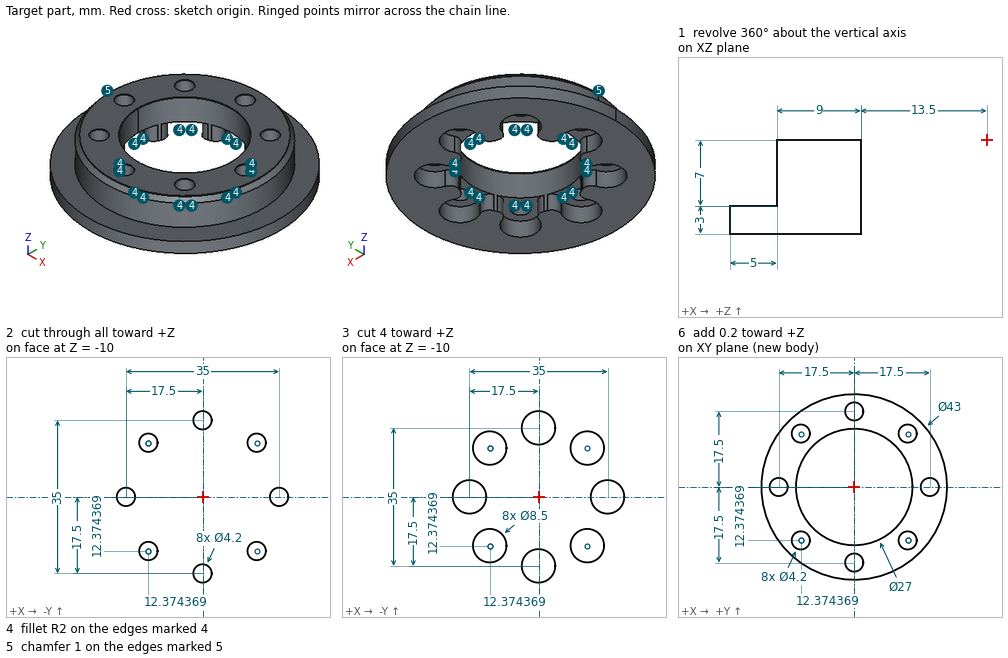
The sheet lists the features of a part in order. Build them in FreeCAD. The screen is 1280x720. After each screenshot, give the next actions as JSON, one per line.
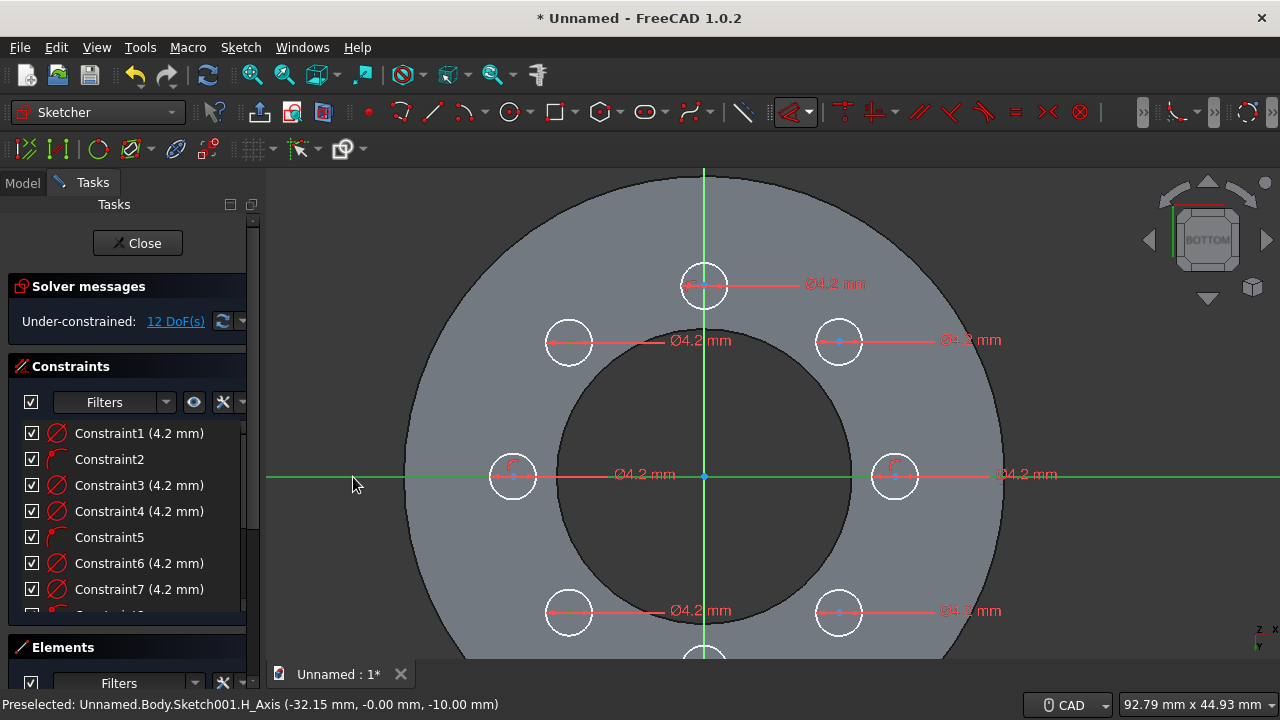
{"action": "key", "text": "s"}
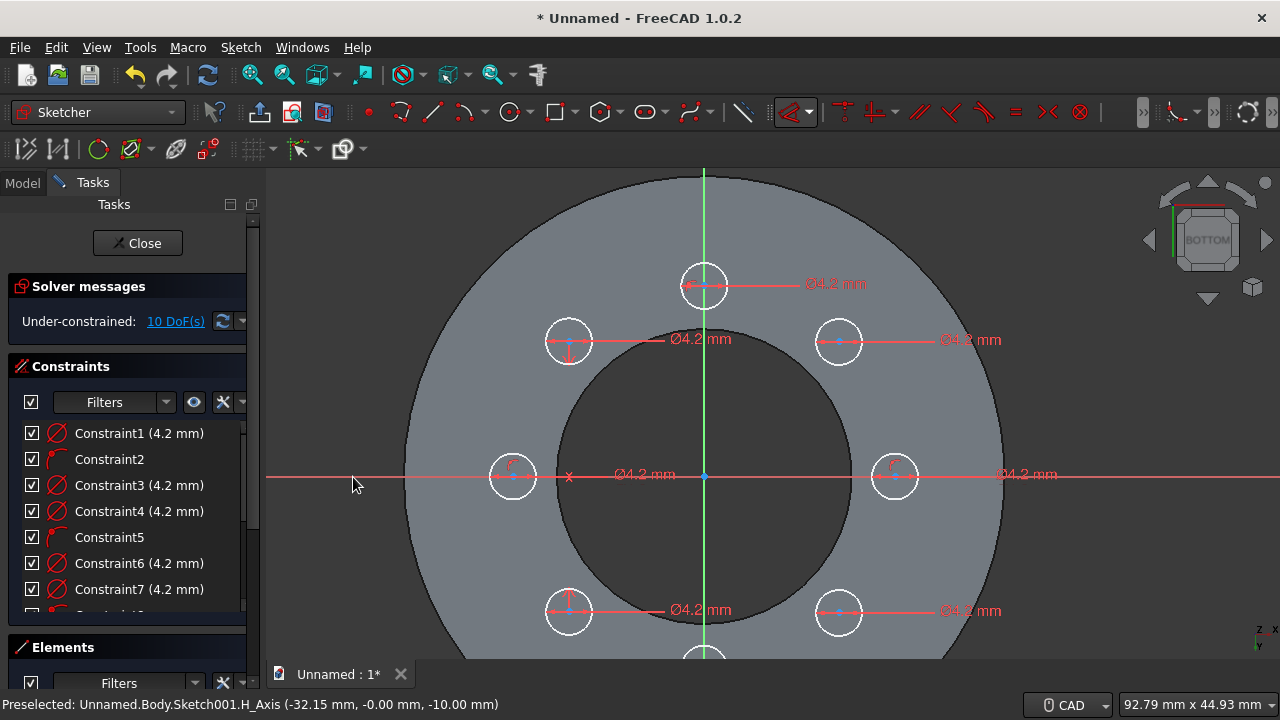
{"action": "left_click", "coordinate": [569, 341]}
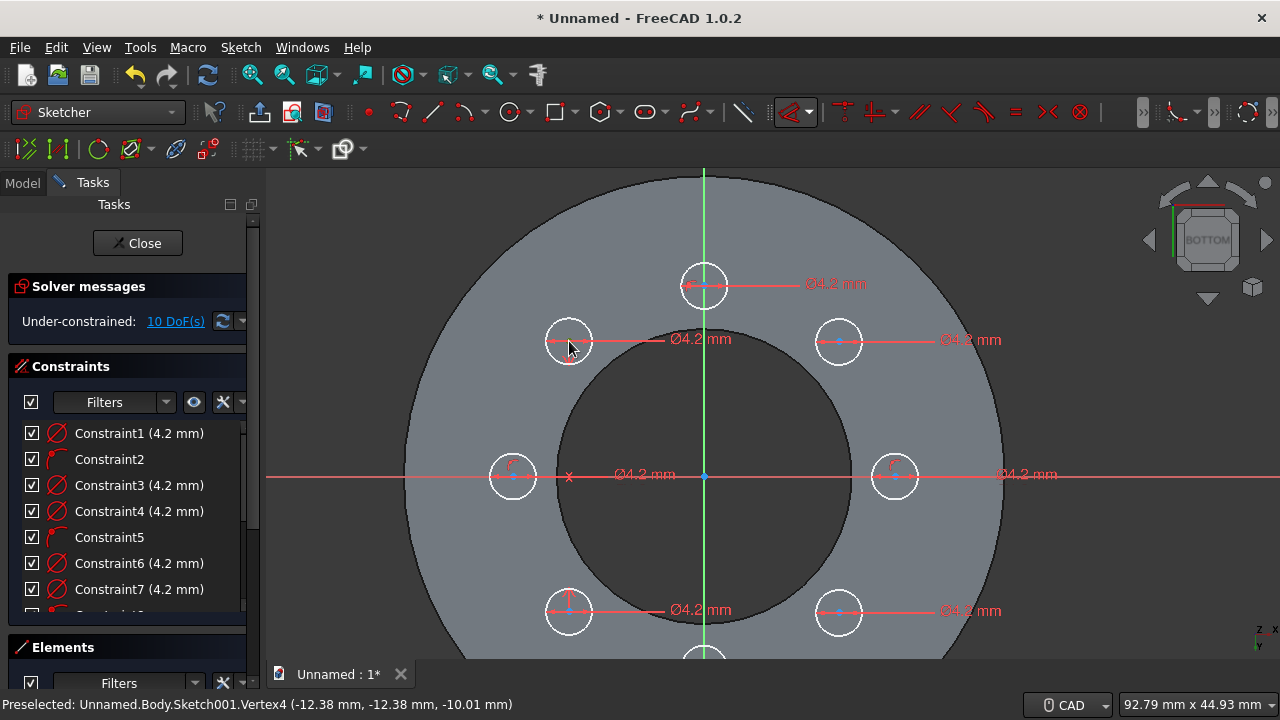
{"action": "left_click", "coordinate": [839, 342]}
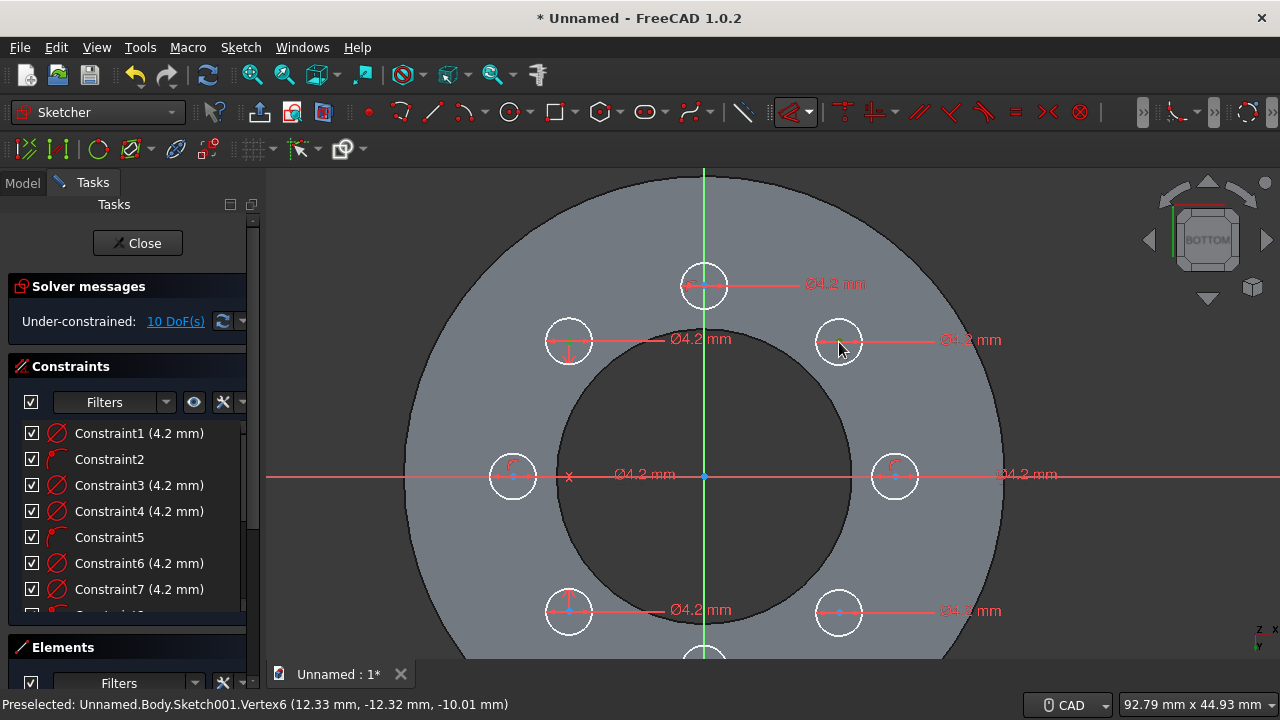
{"action": "left_click", "coordinate": [704, 600]}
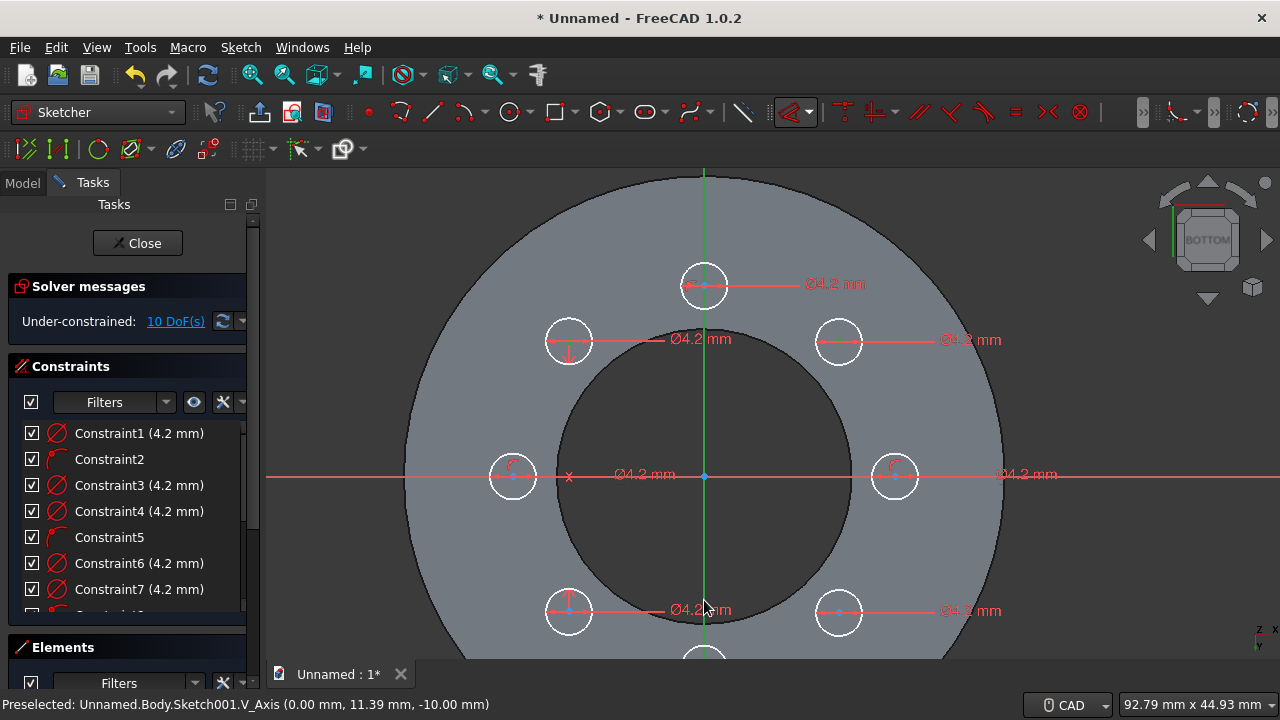
{"action": "key", "text": "s"}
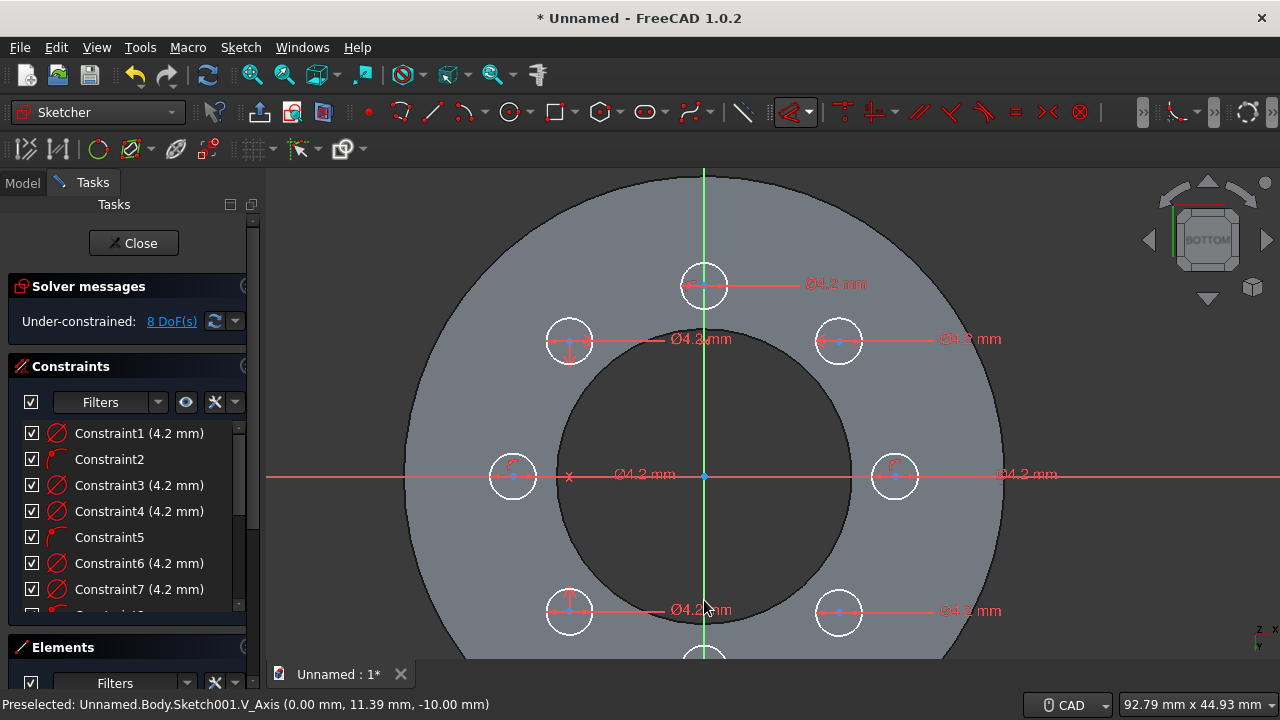
{"action": "left_click", "coordinate": [570, 612]}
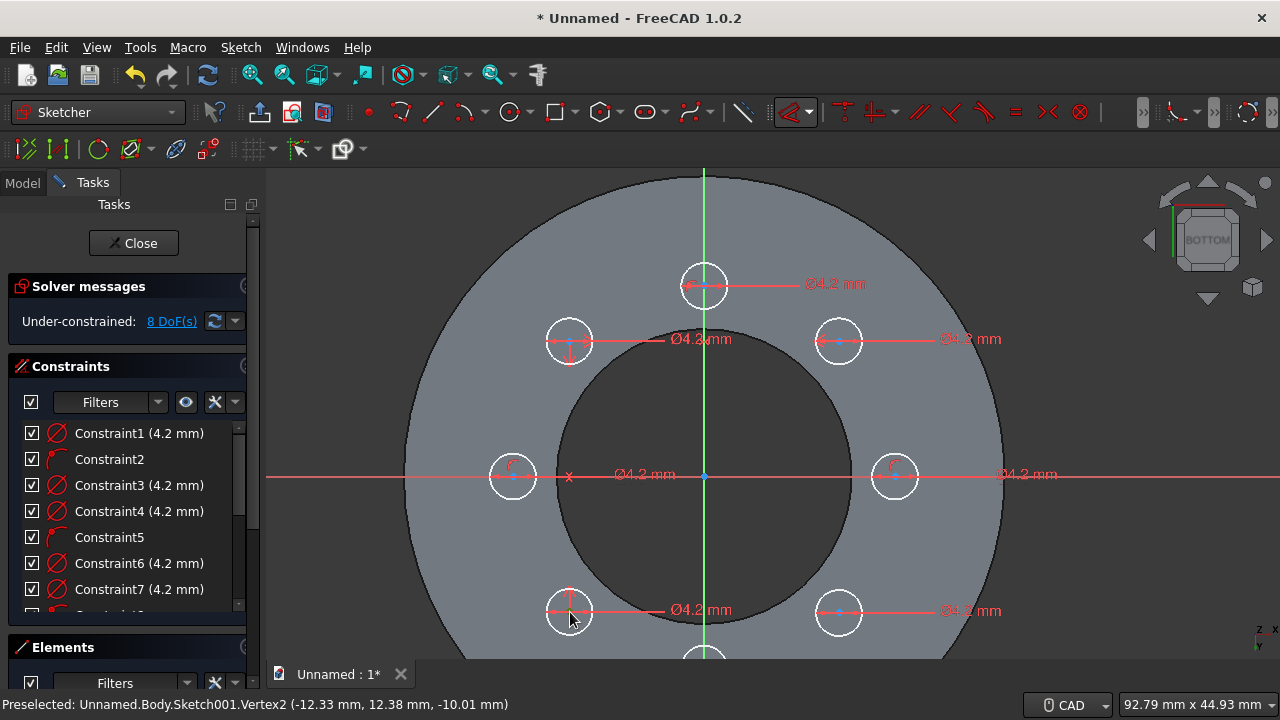
{"action": "left_click", "coordinate": [839, 613]}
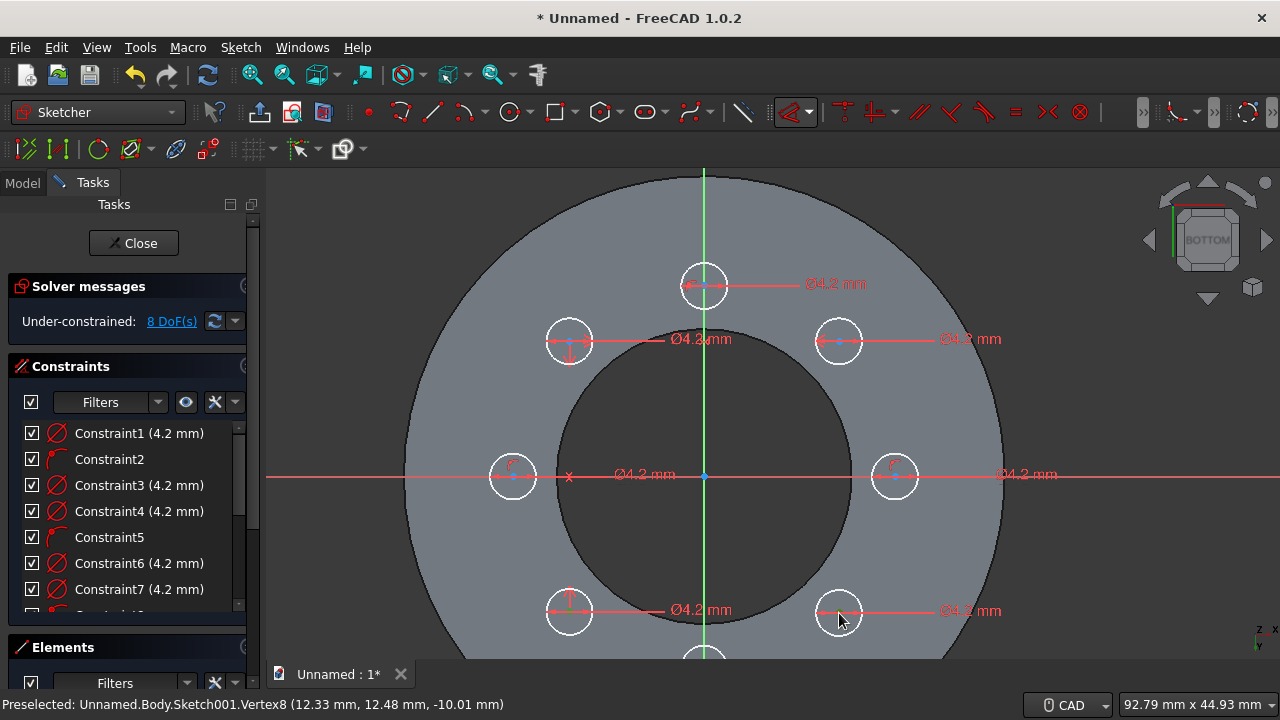
{"action": "left_click", "coordinate": [704, 600]}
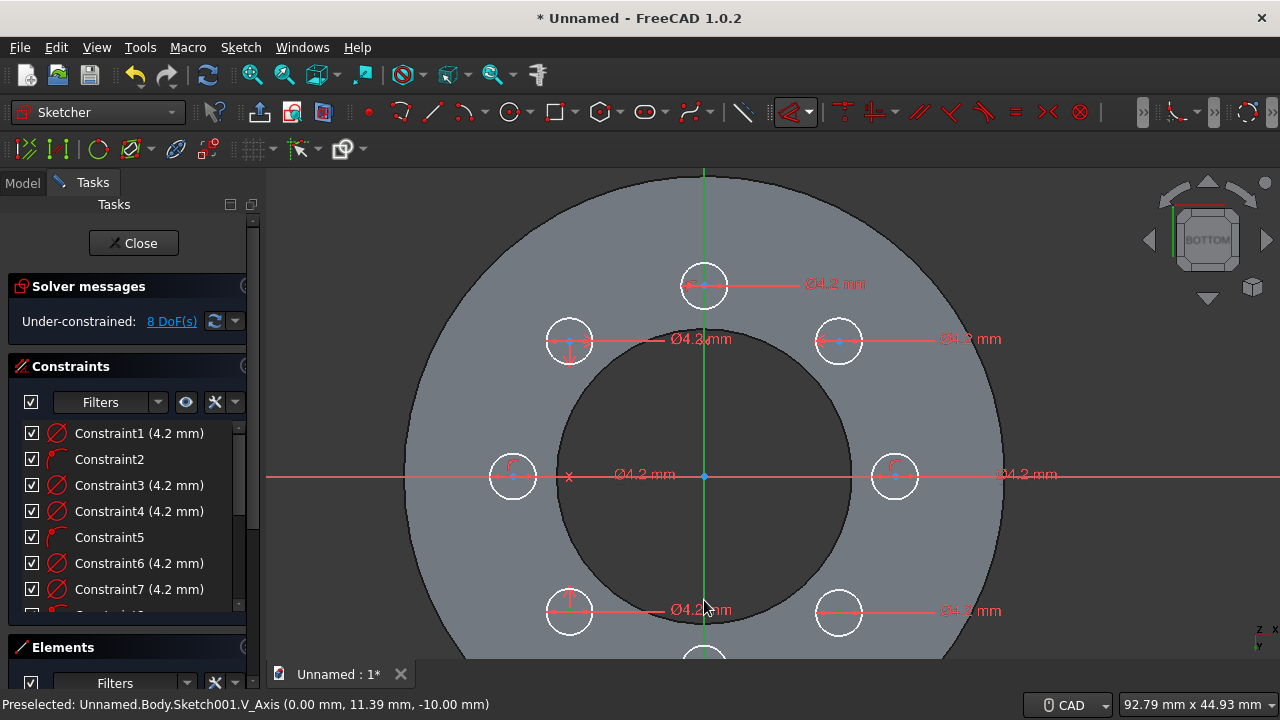
{"action": "key", "text": "s"}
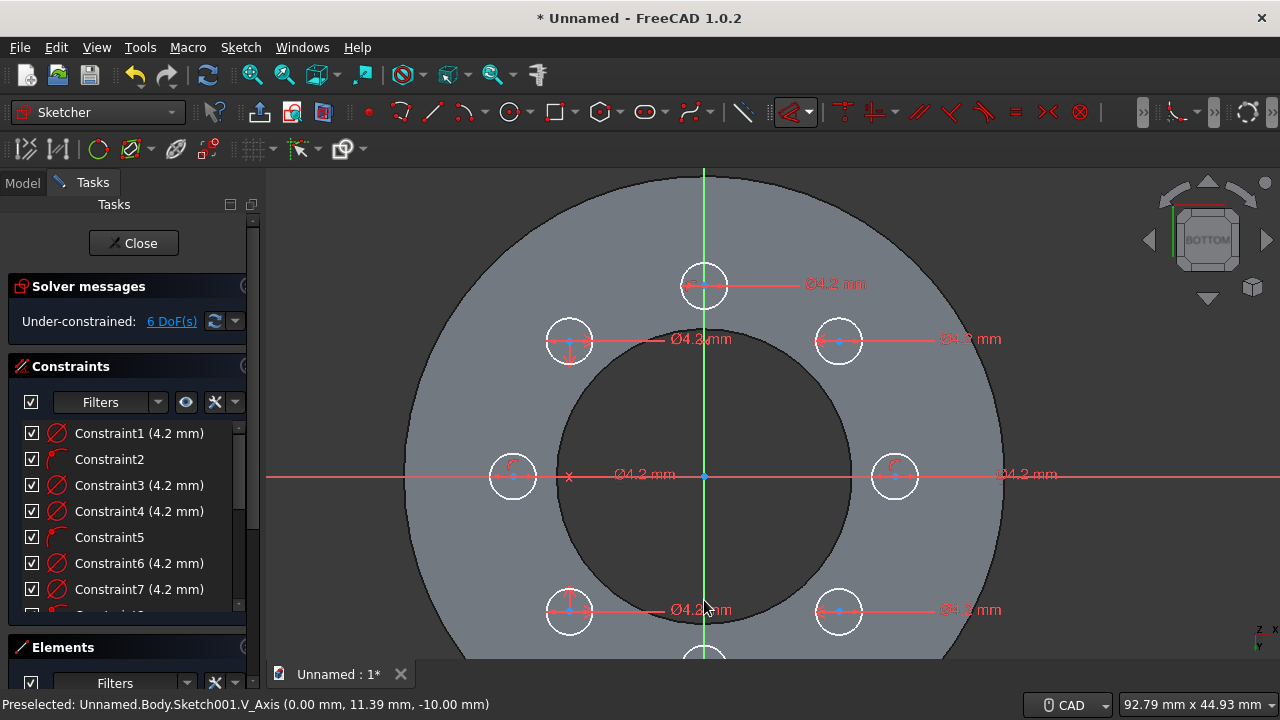
{"action": "scroll", "coordinate": [705, 285], "scroll_direction": "down", "scroll_amount": 2}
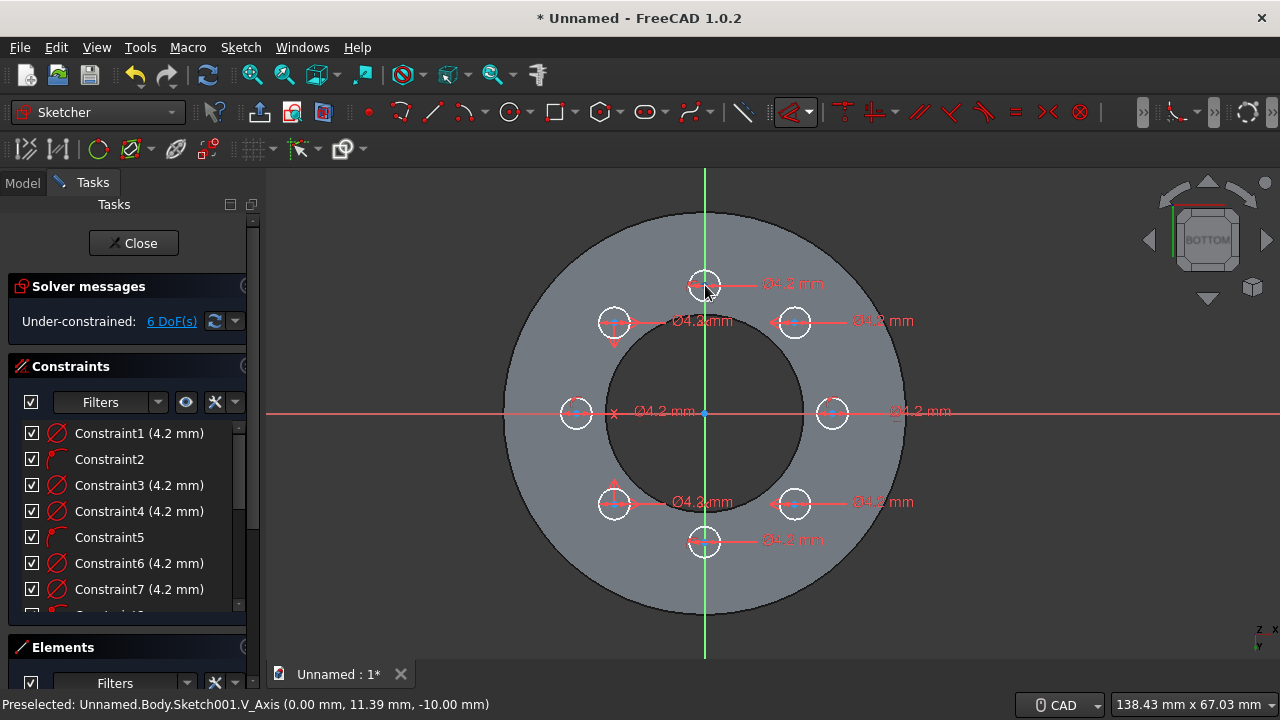
{"action": "left_click", "coordinate": [705, 542]}